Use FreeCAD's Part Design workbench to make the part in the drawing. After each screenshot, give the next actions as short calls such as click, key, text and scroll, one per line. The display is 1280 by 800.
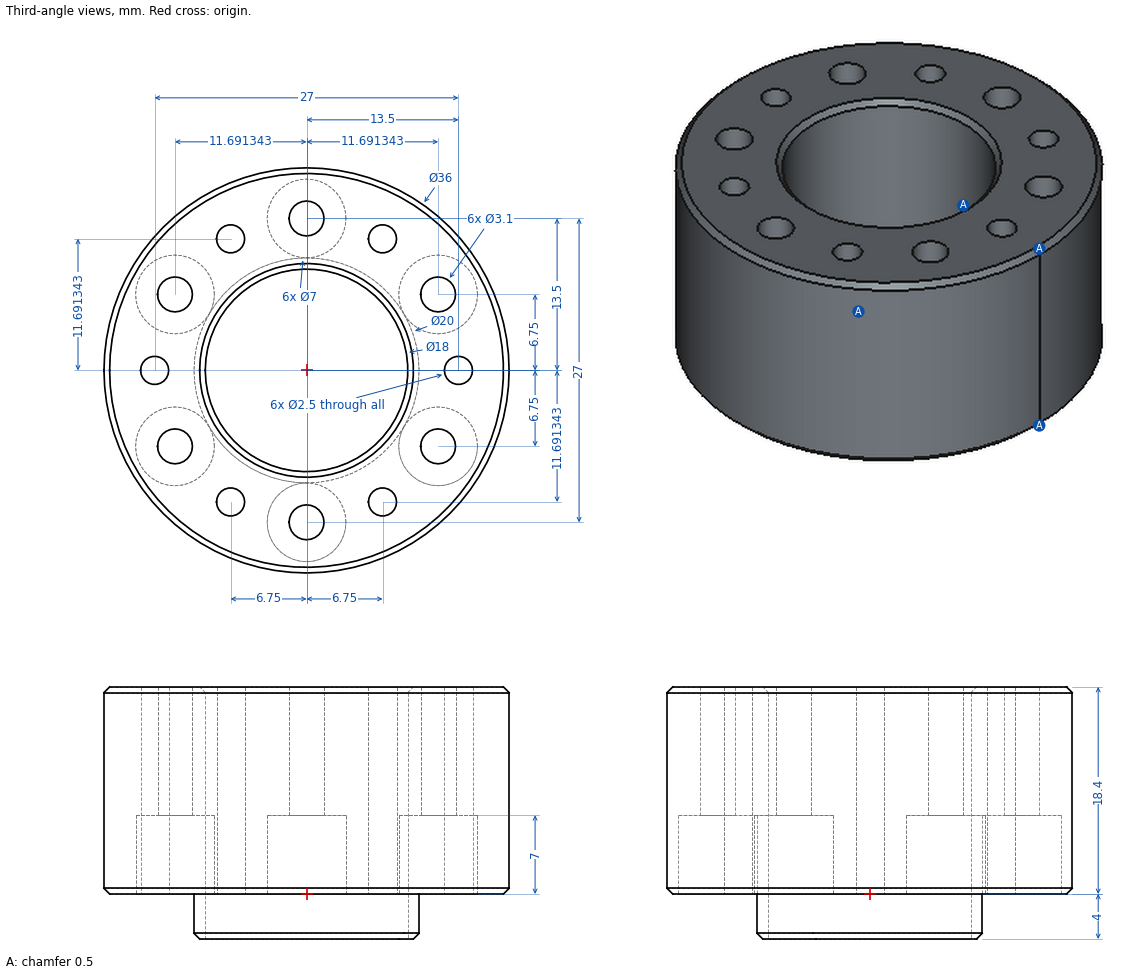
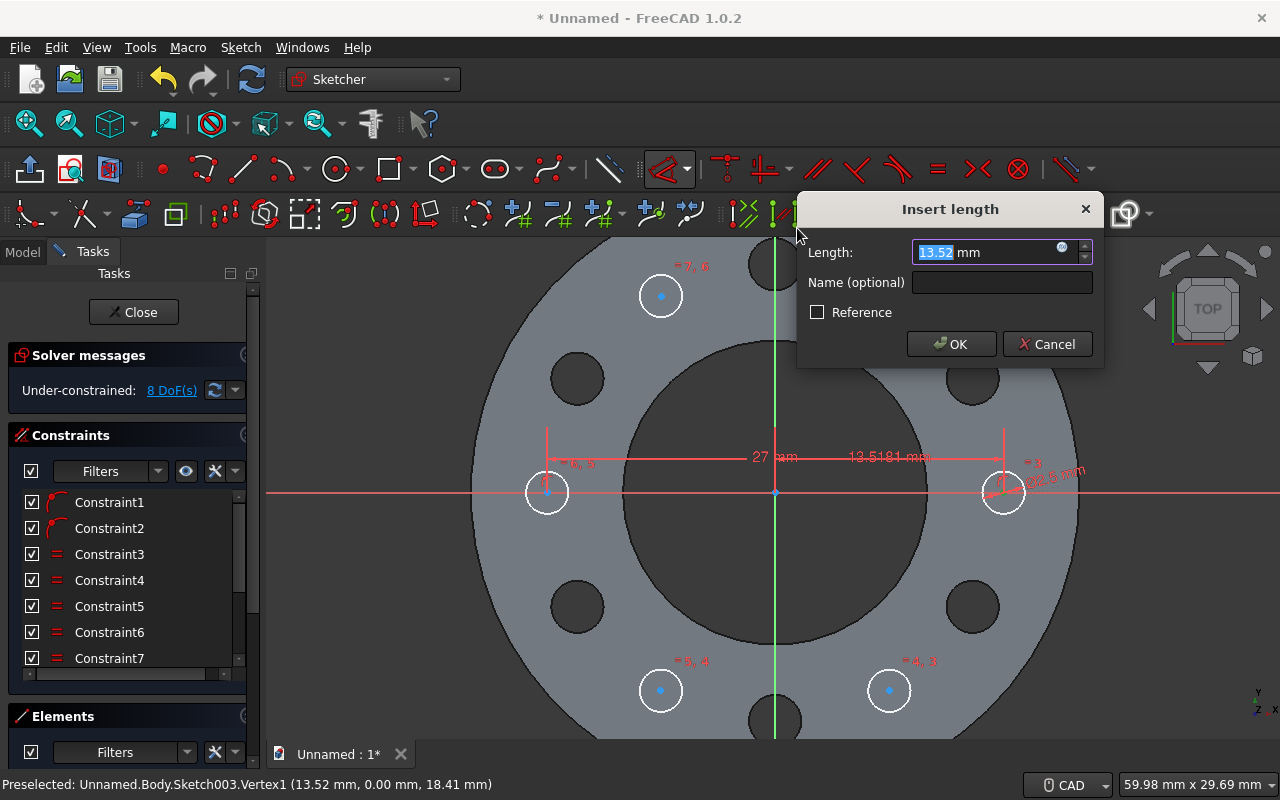
text(13.5)
key(Return)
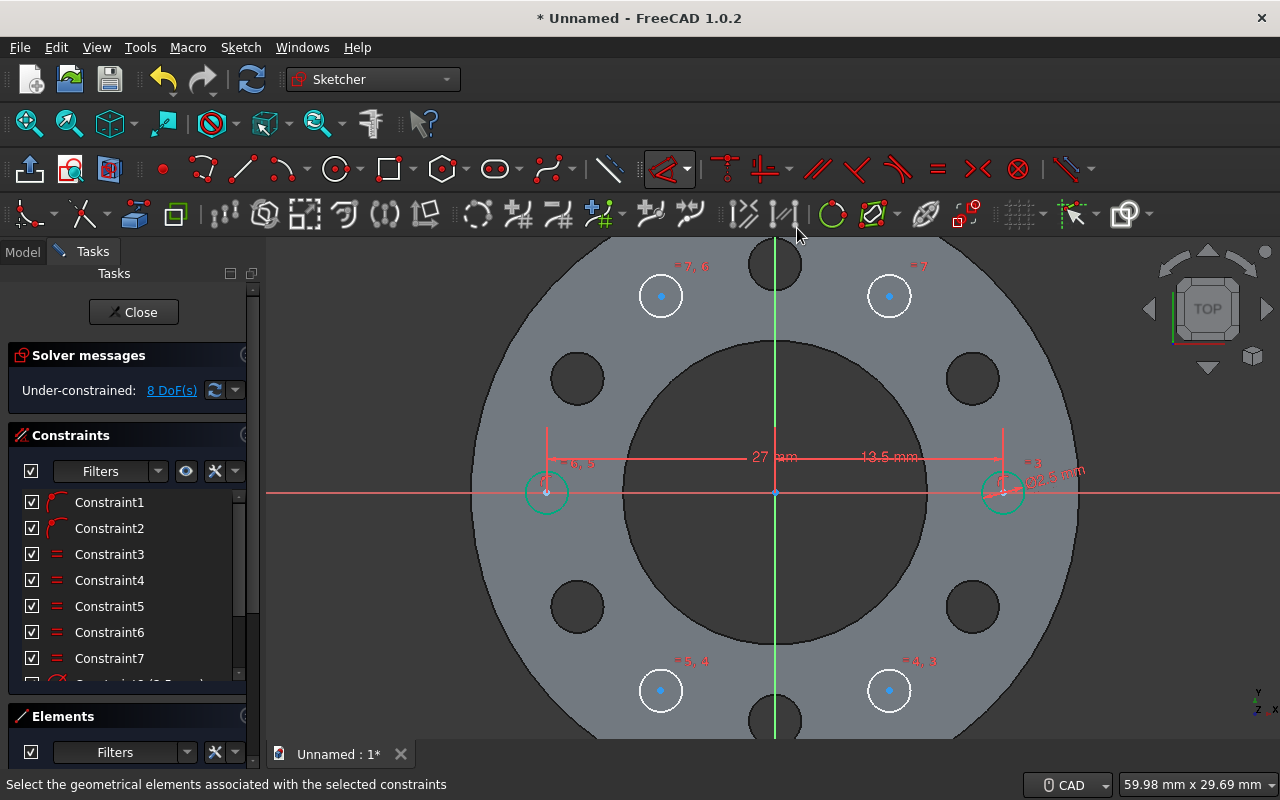
click(889, 691)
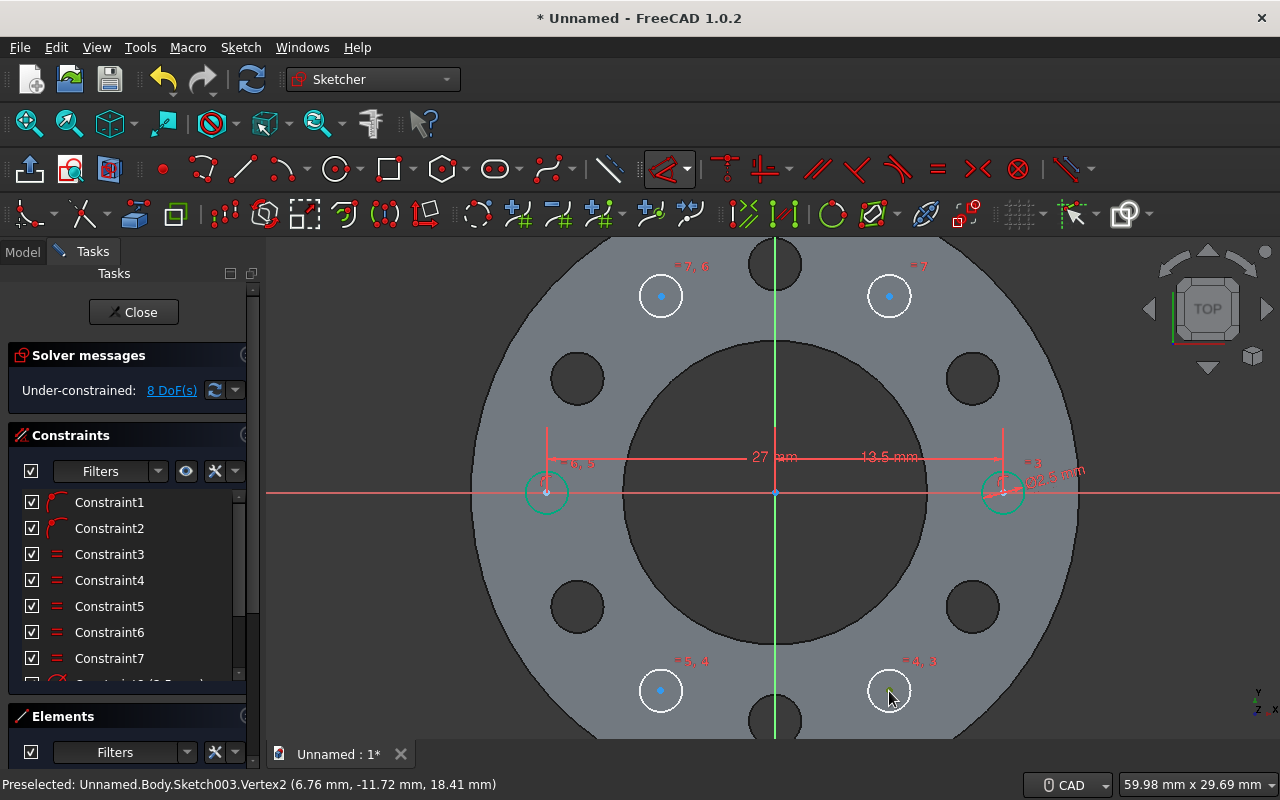
key(l)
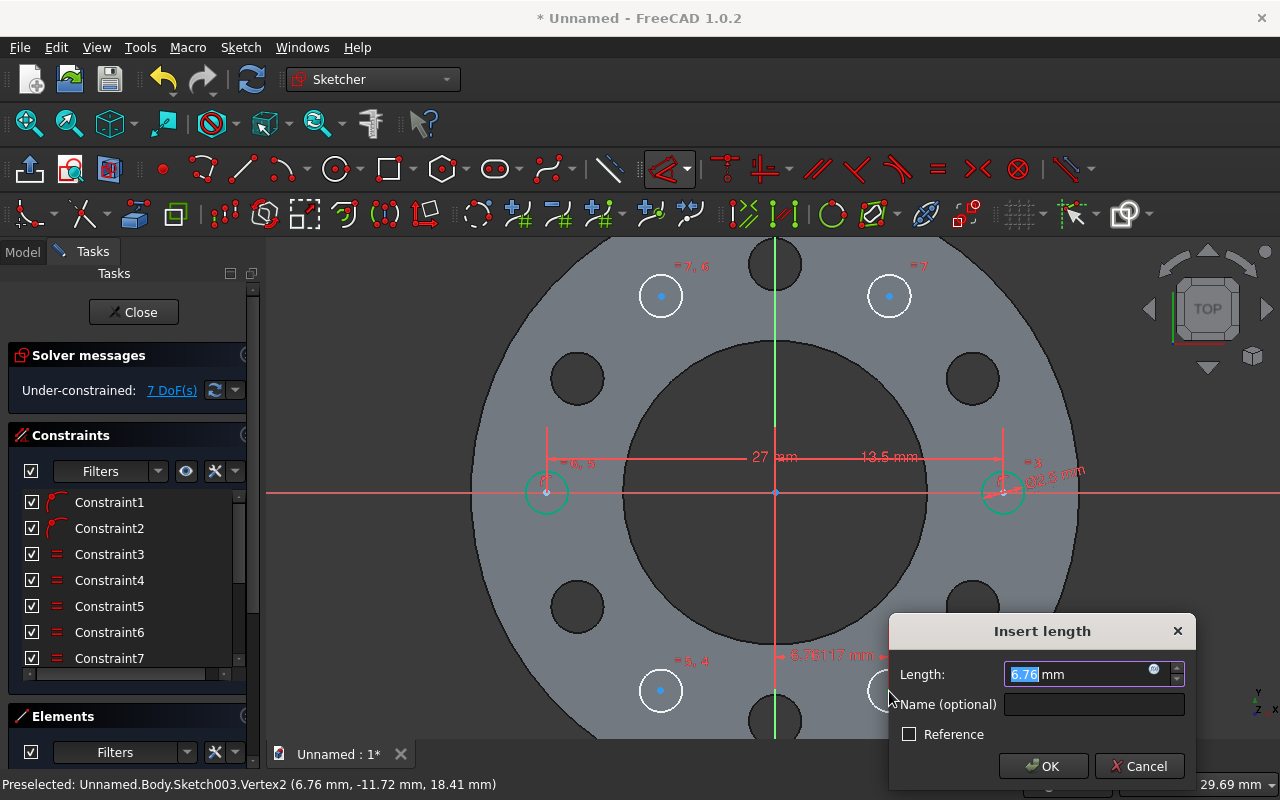
text(6.75)
key(Return)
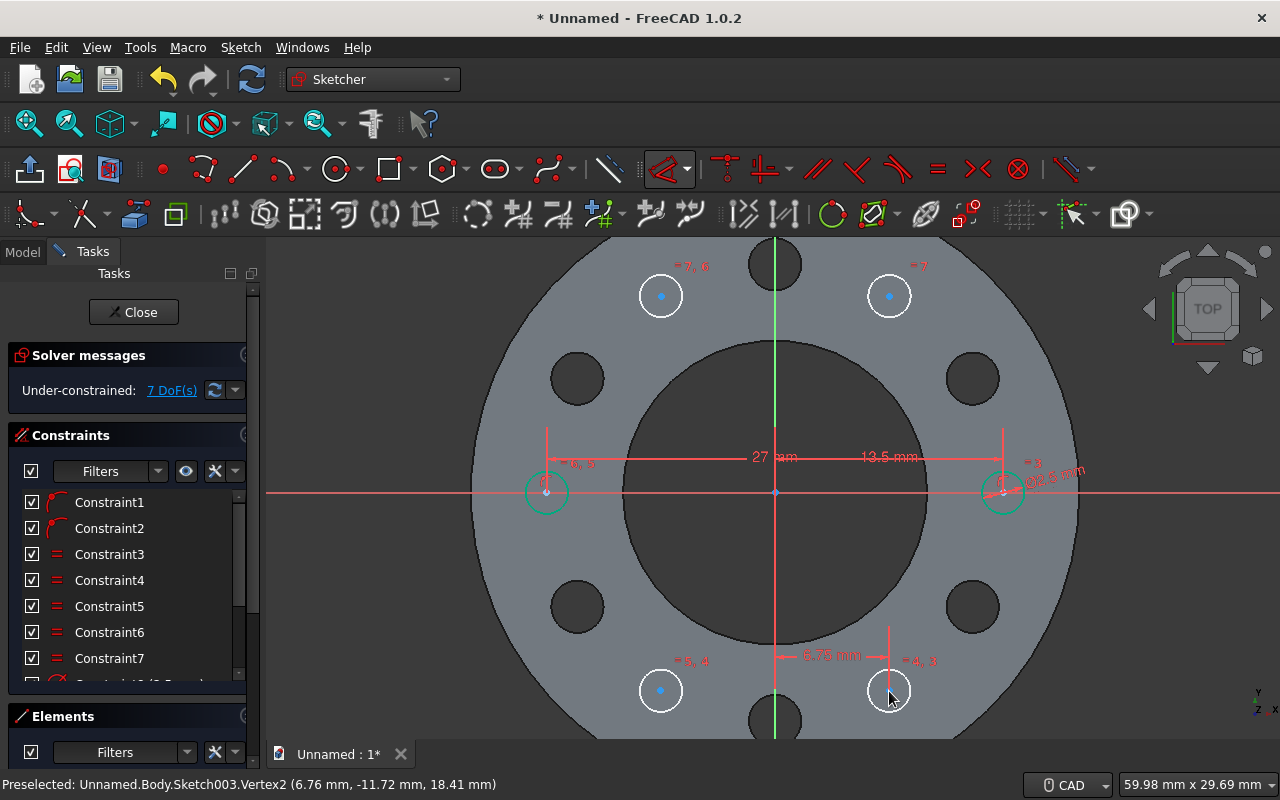
click(661, 691)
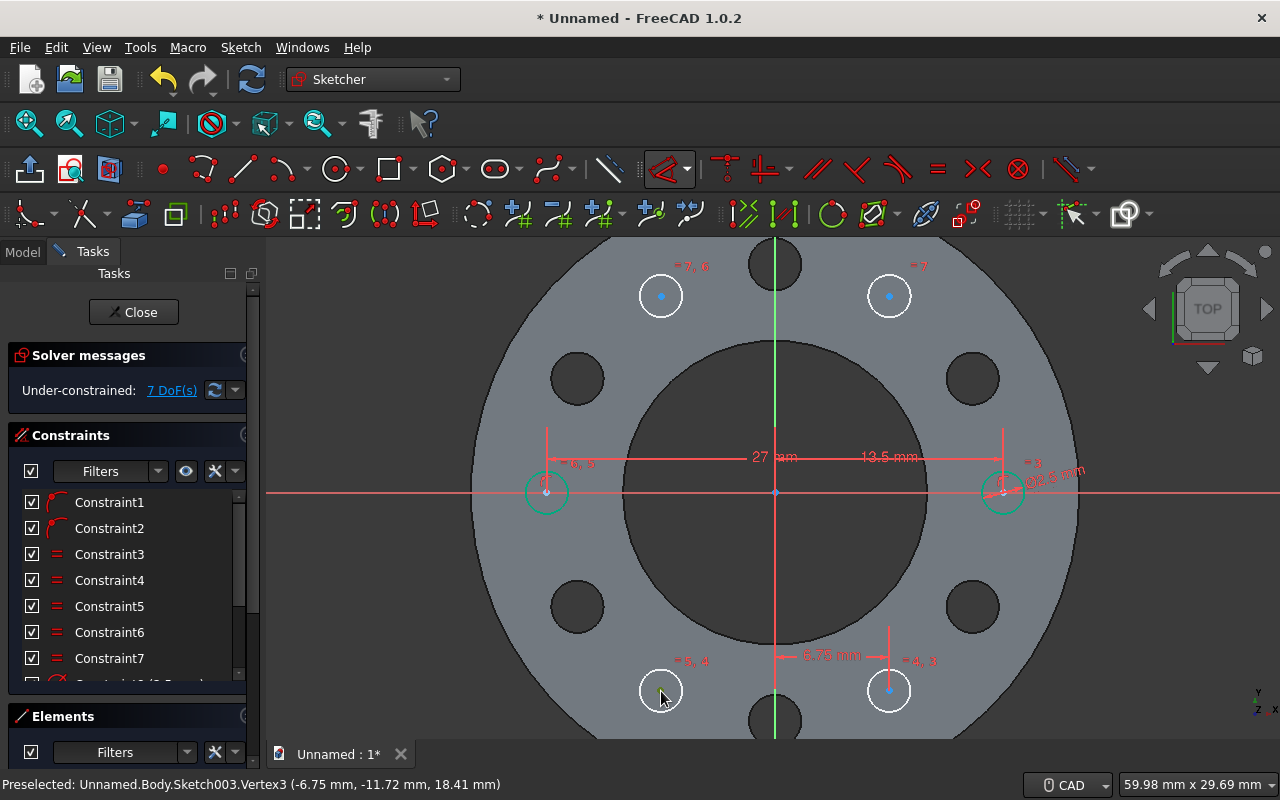
click(690, 170)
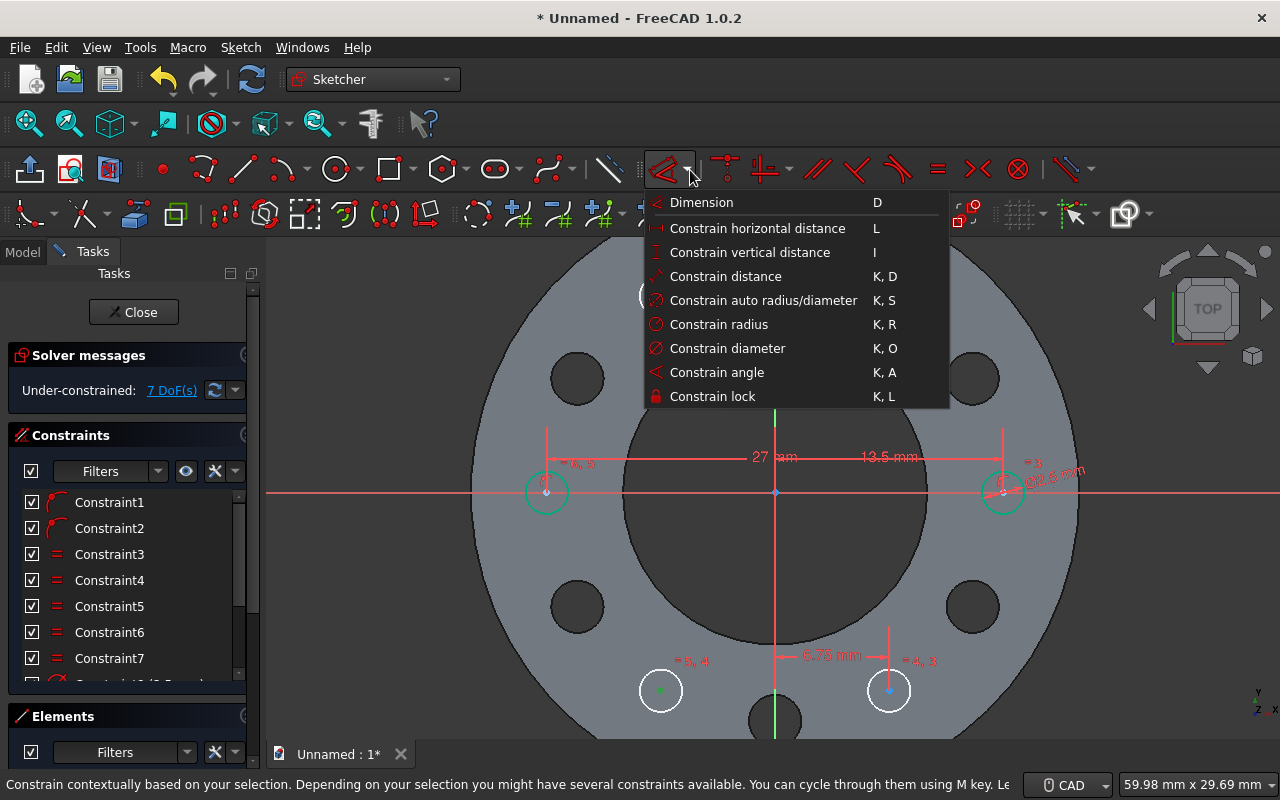
click(797, 228)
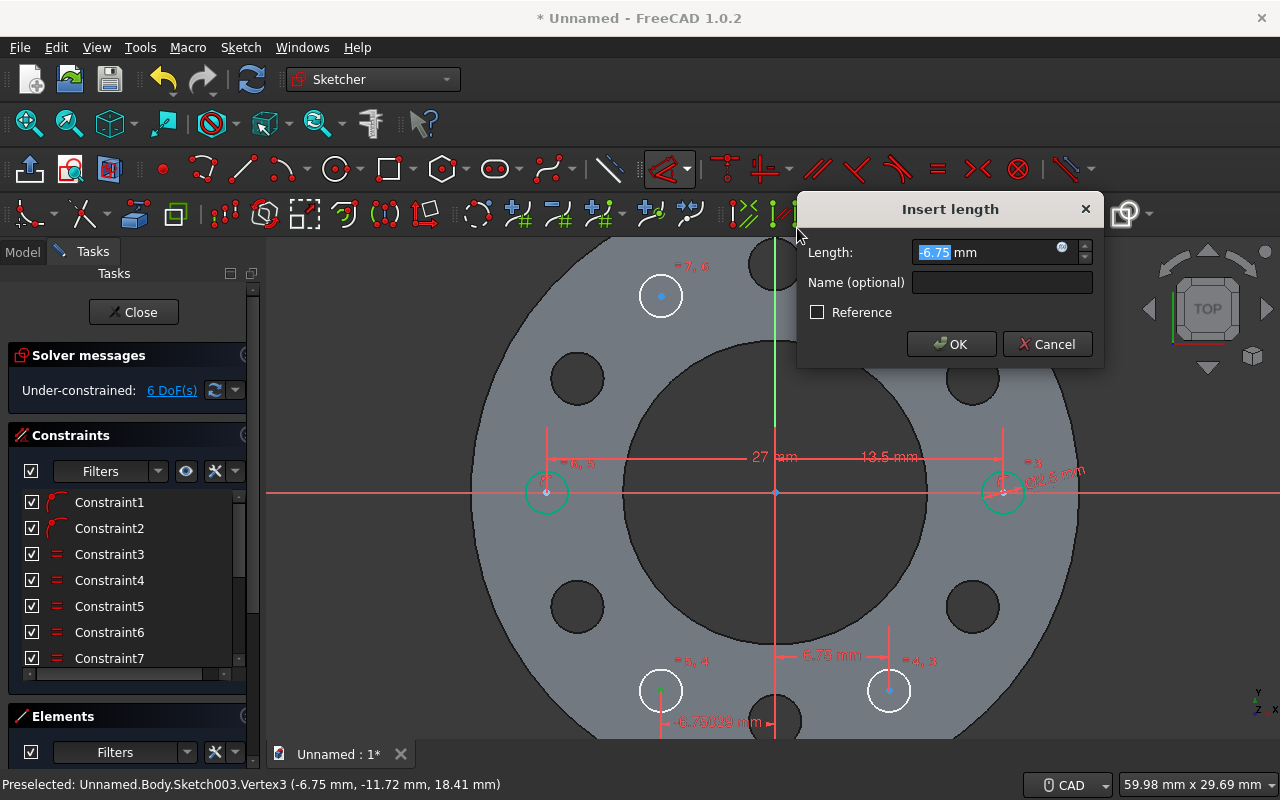
text(-6.75)
key(Return)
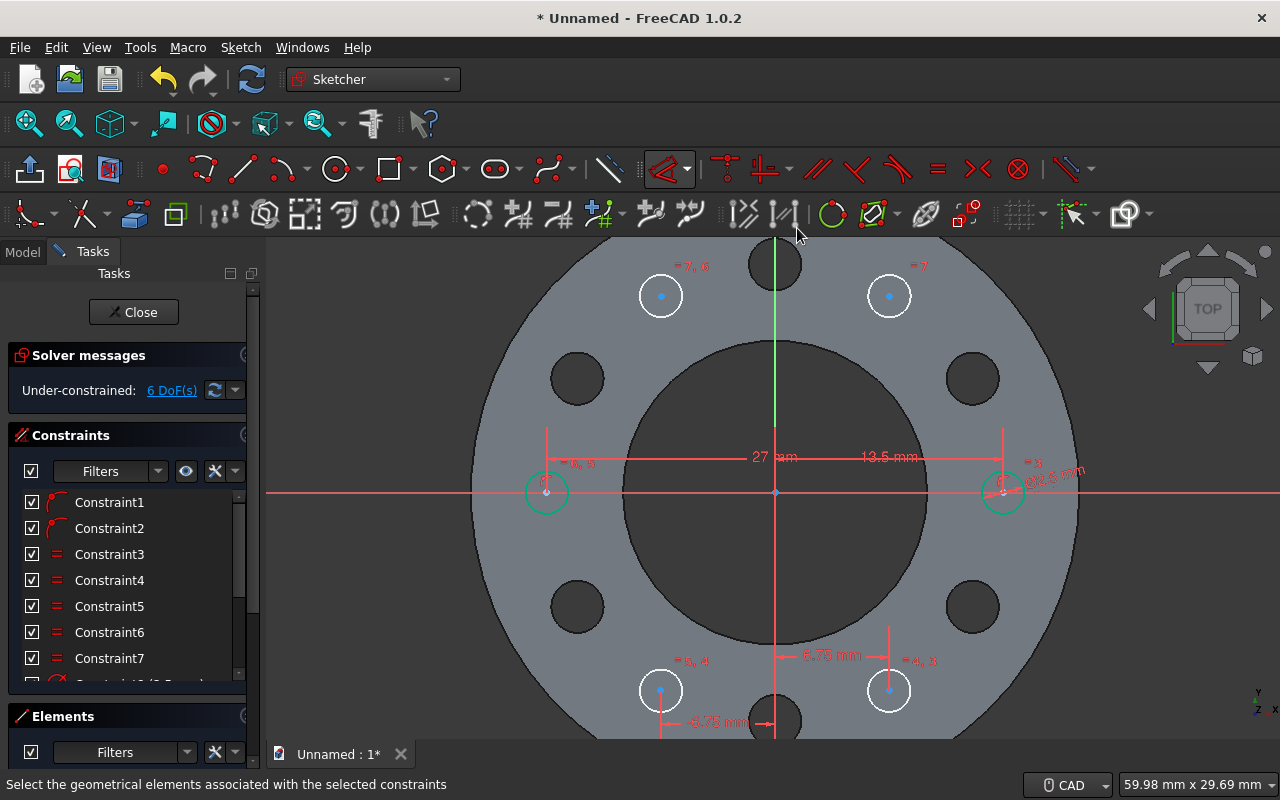
click(661, 296)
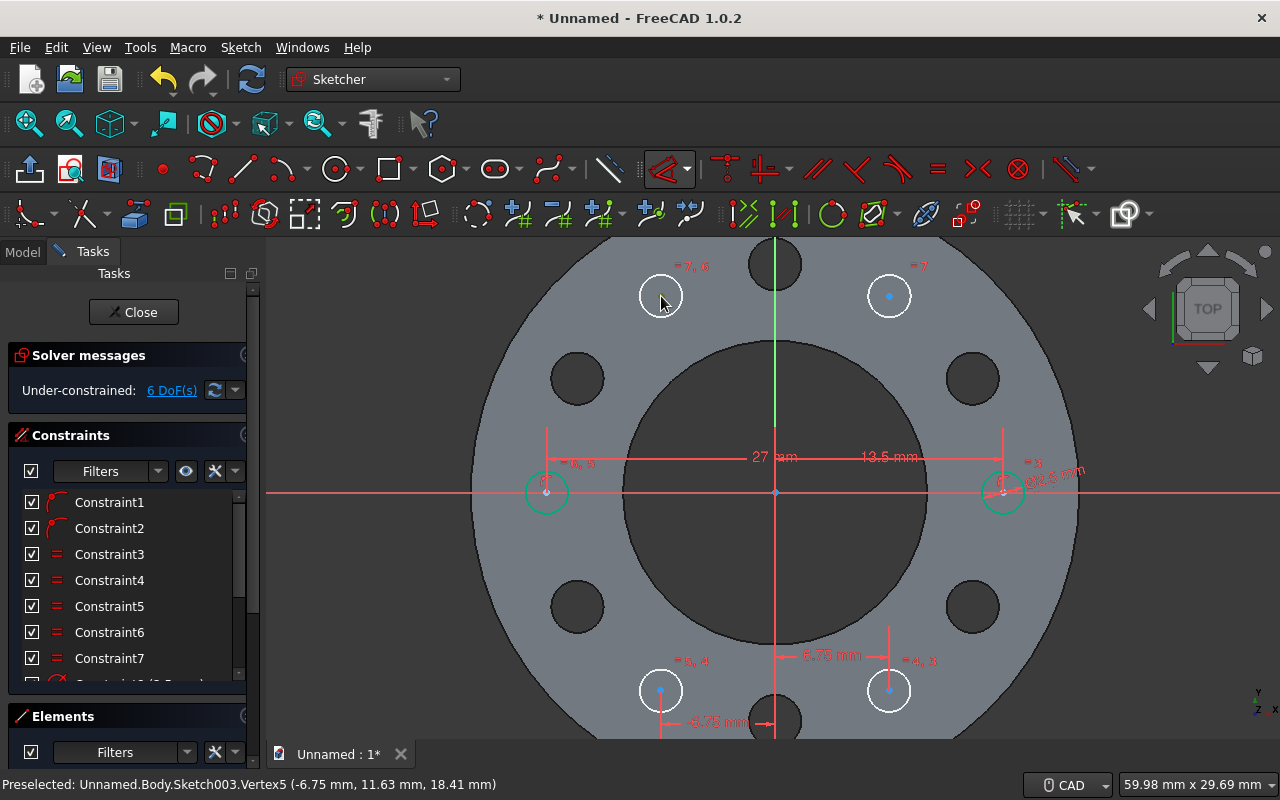
click(690, 170)